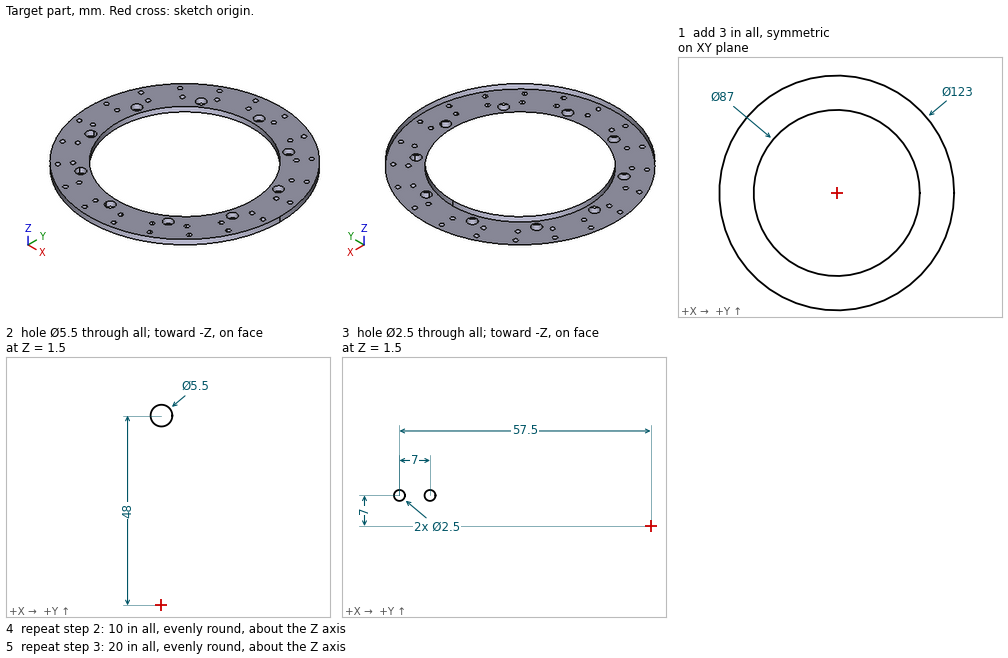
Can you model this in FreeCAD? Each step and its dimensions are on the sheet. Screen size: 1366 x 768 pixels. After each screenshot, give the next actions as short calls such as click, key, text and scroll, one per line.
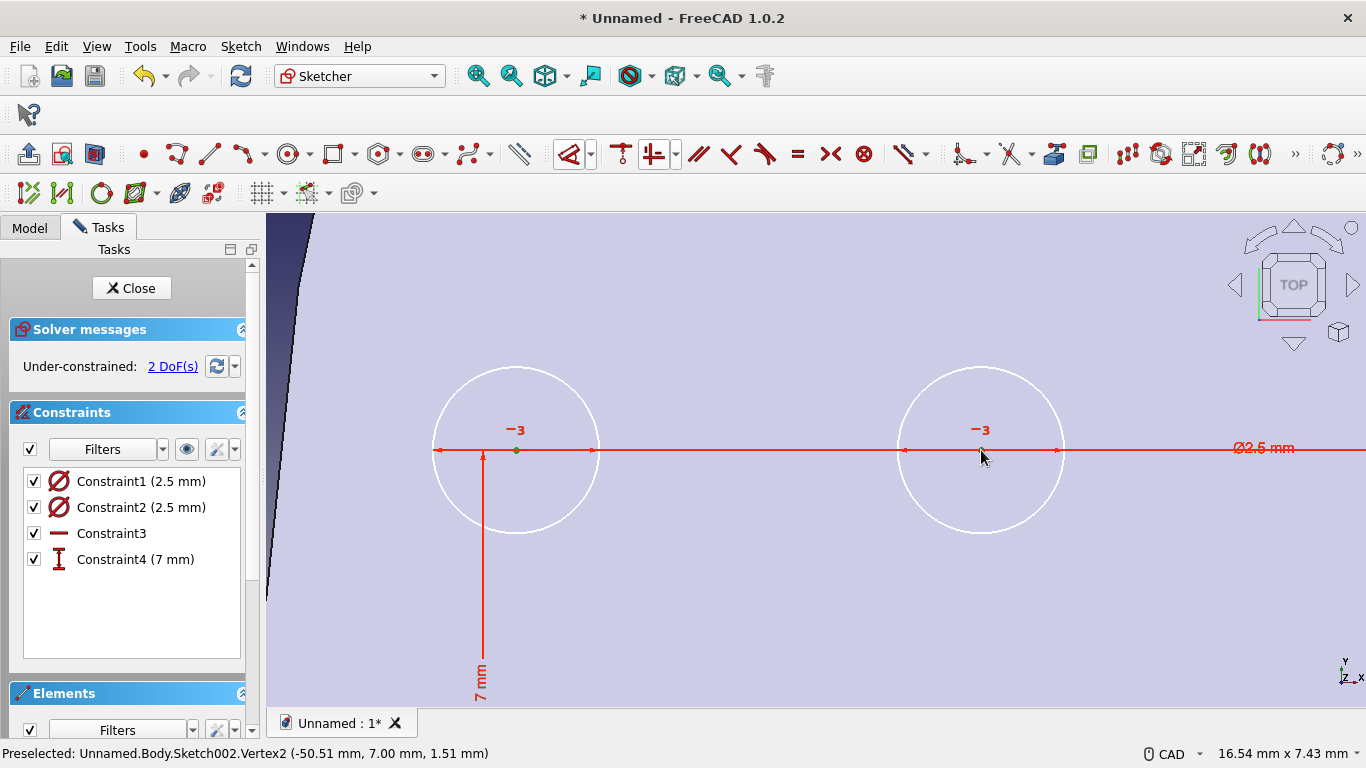
click(590, 154)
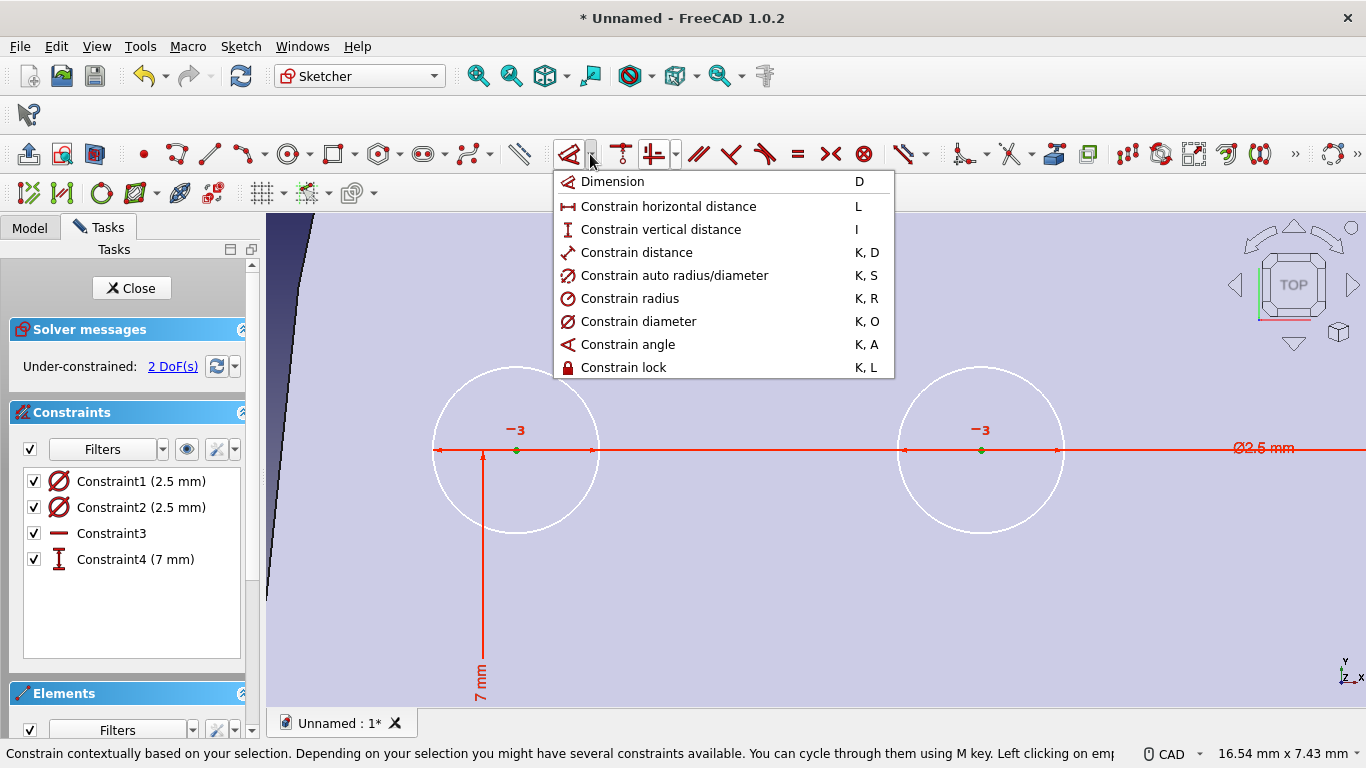
click(724, 206)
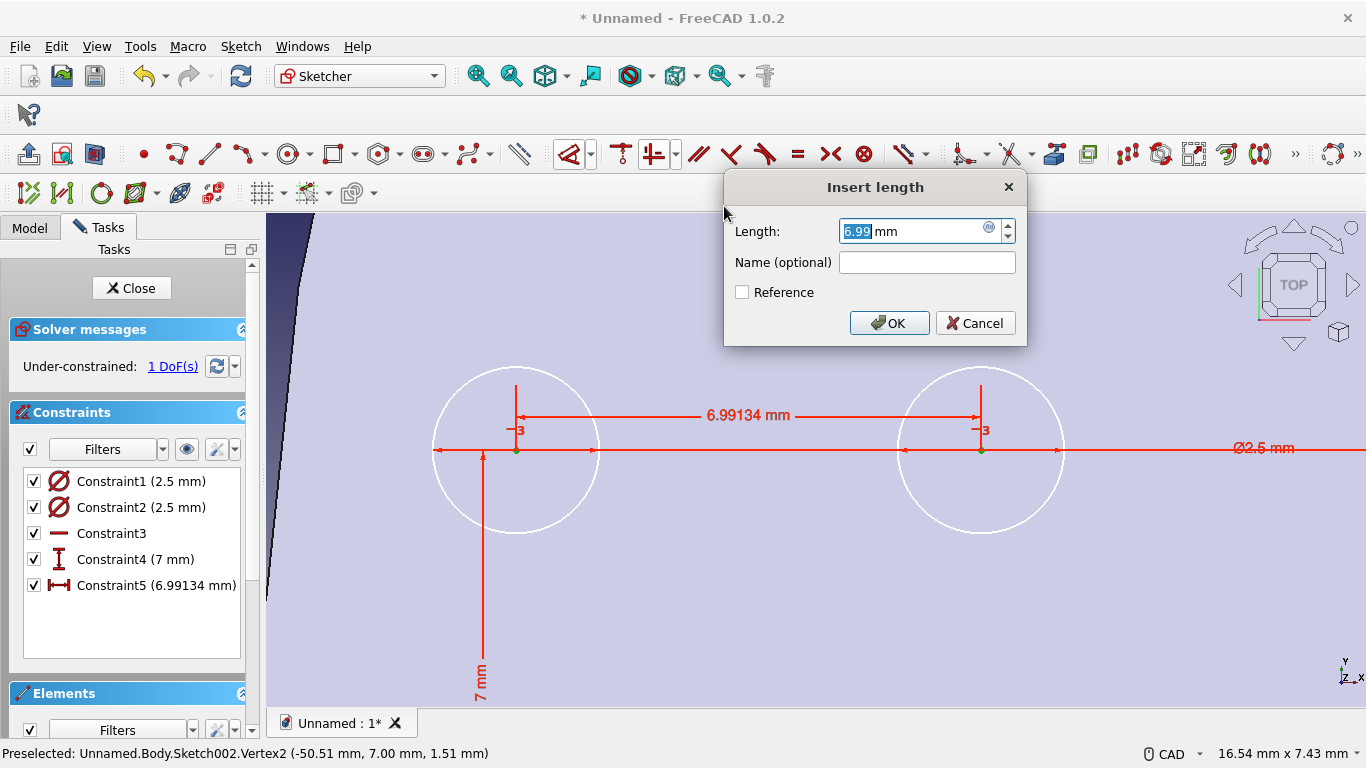
text(7)
key(Return)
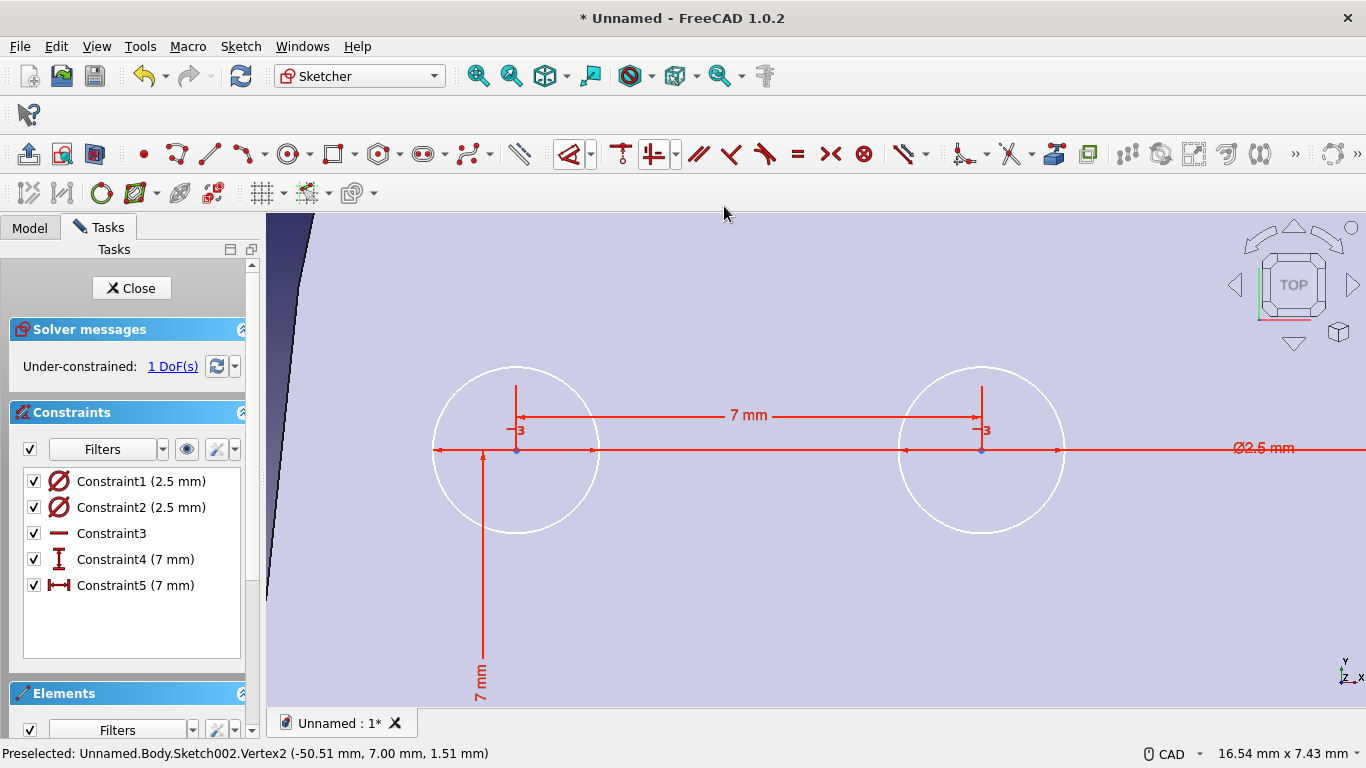
click(516, 450)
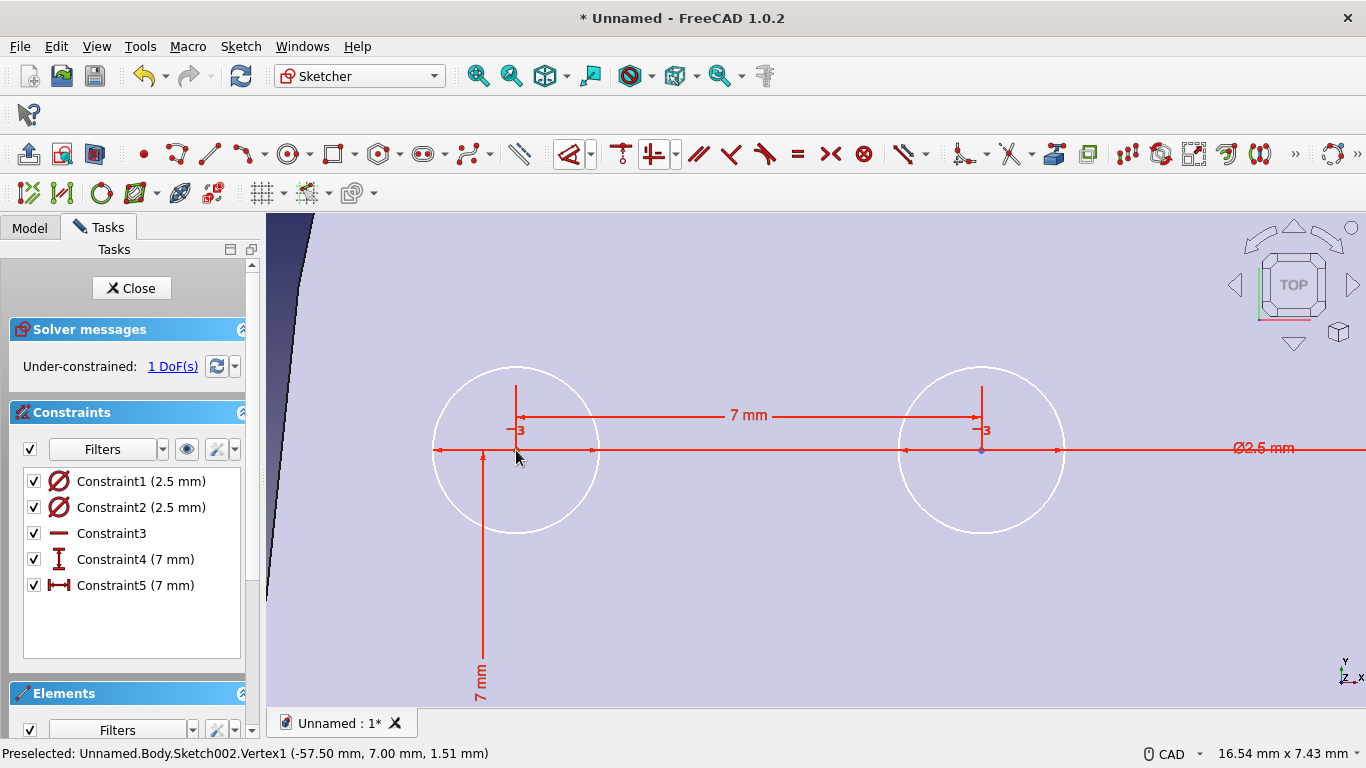
key(l)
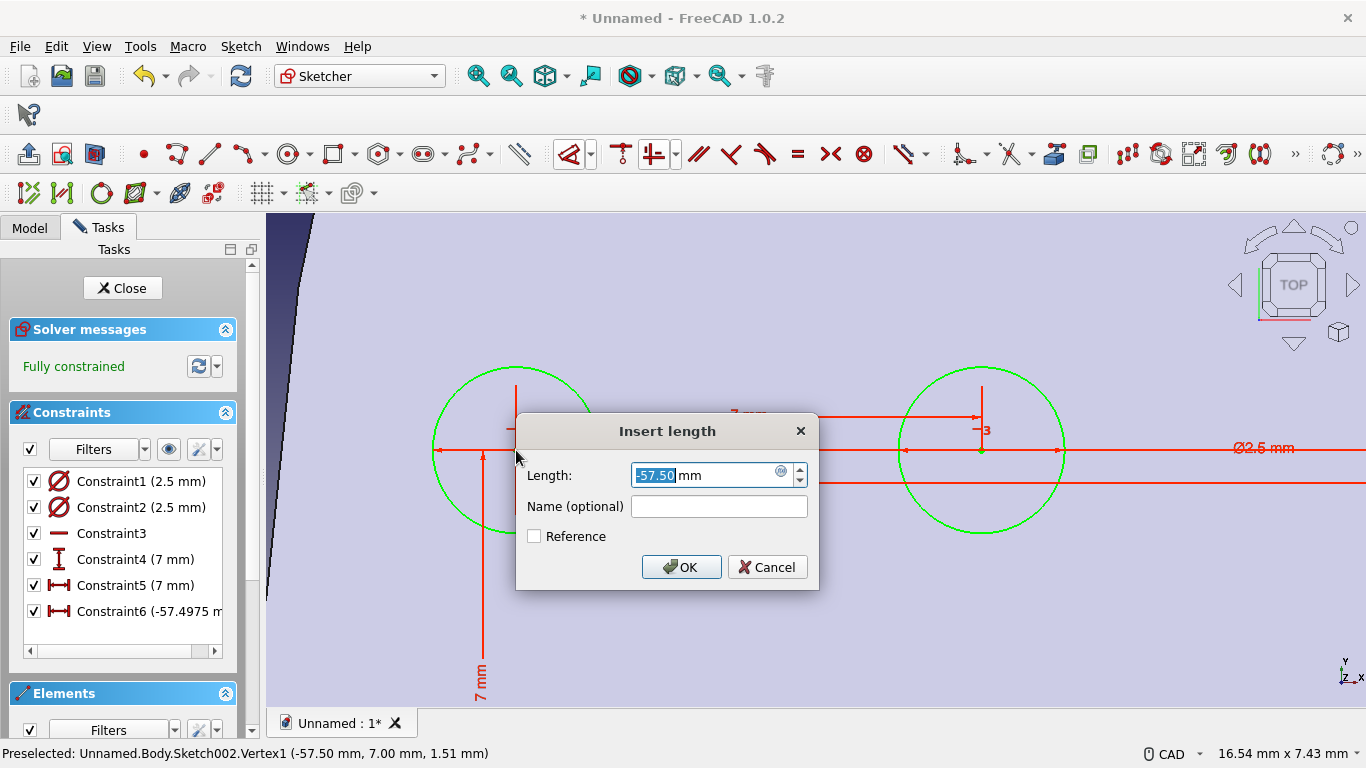
text(-57.5)
key(Return)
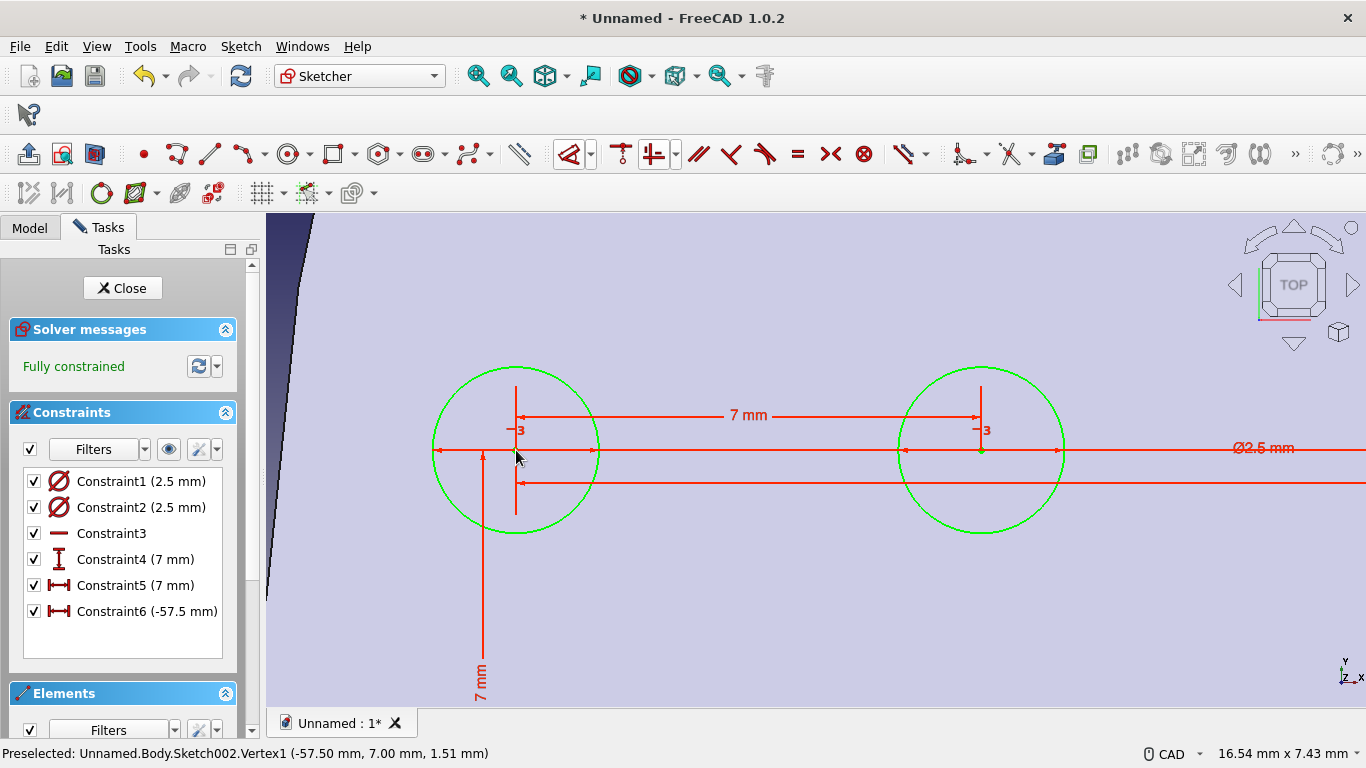
click(123, 288)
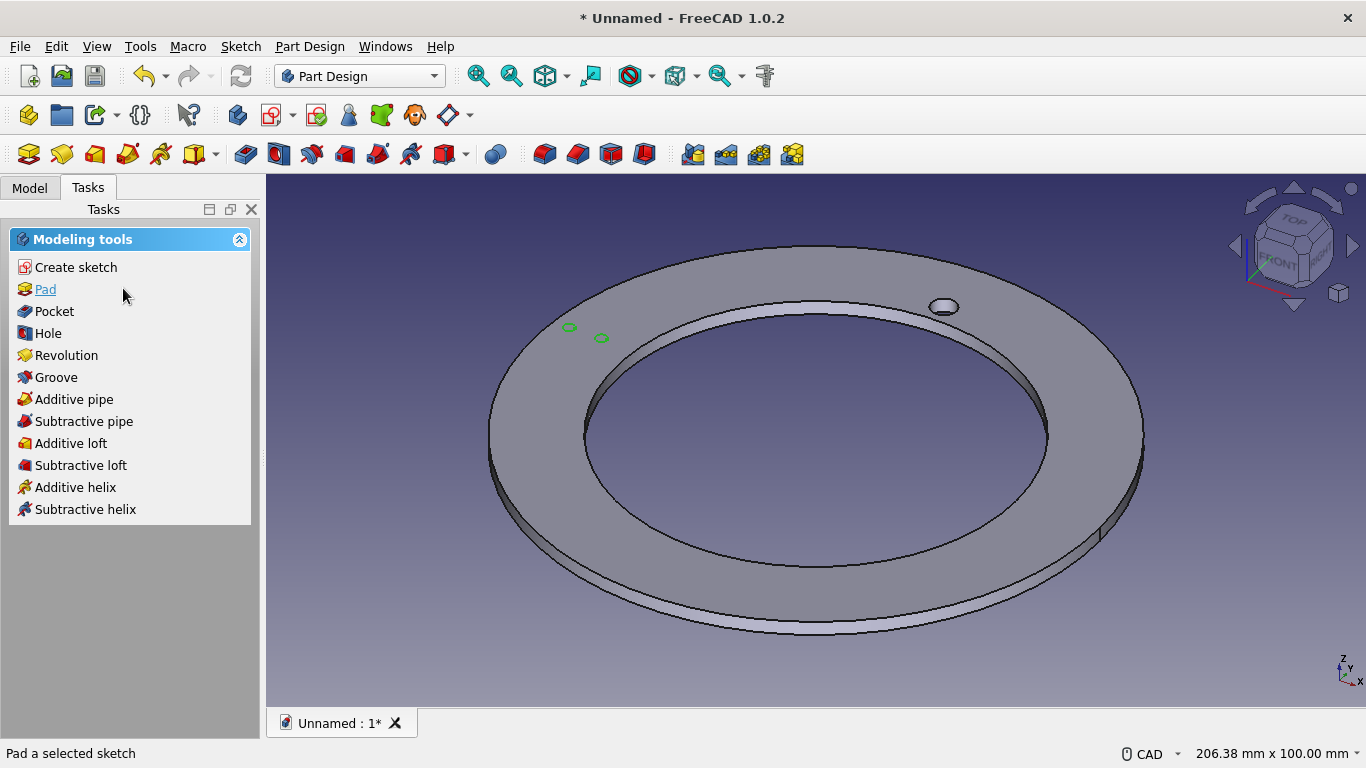
click(279, 154)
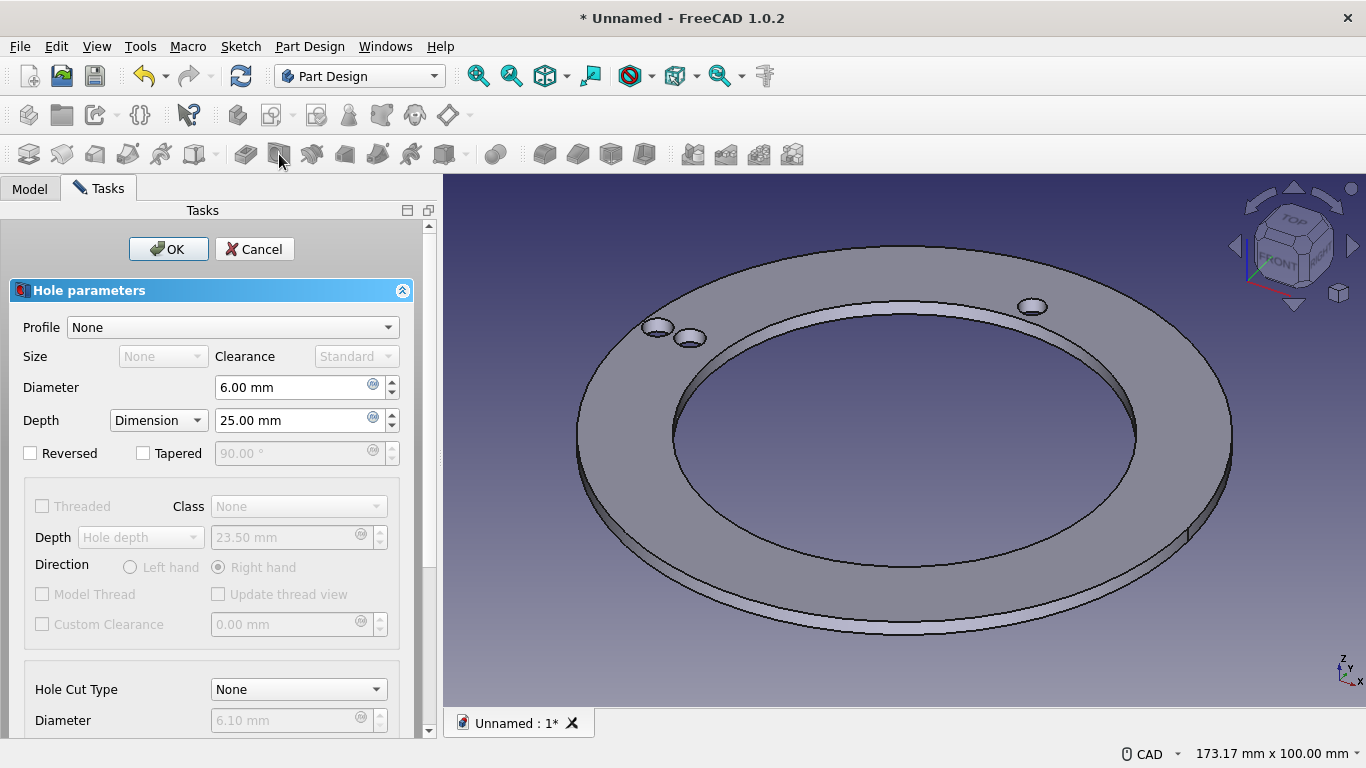
triple_click(300, 388)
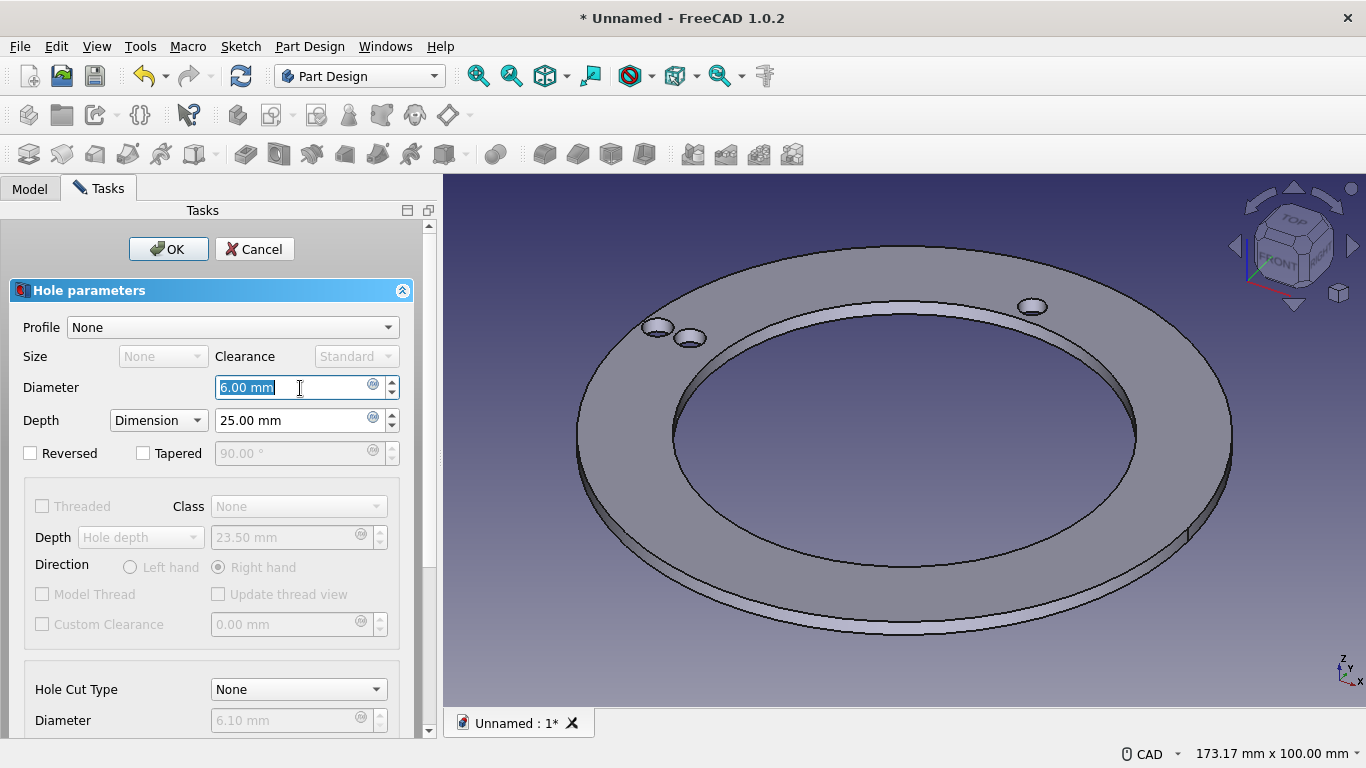
text(2.5)
key(Tab)